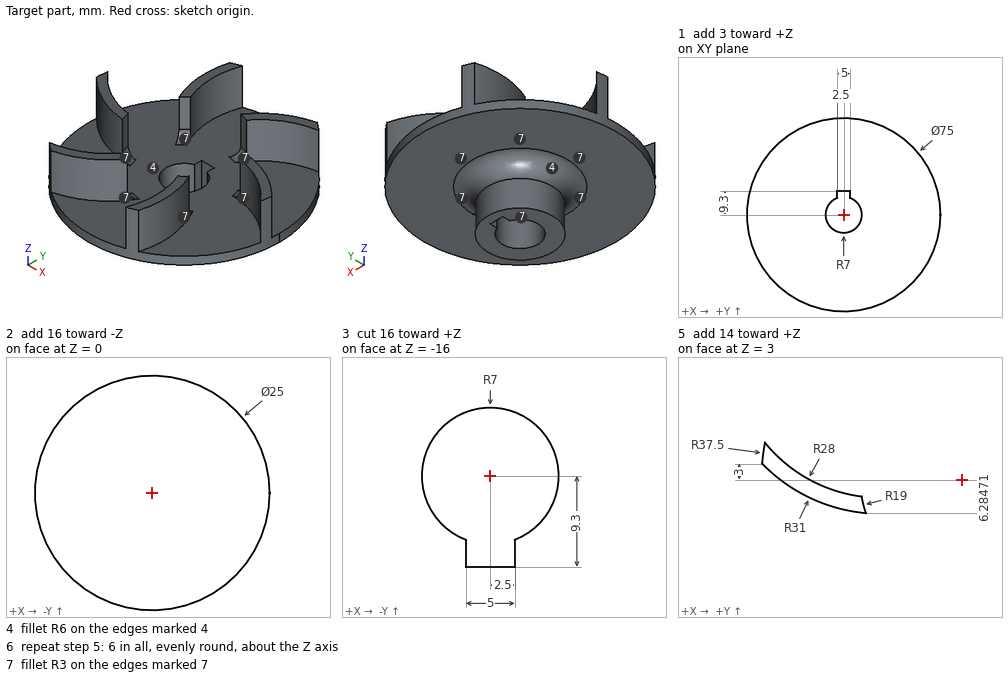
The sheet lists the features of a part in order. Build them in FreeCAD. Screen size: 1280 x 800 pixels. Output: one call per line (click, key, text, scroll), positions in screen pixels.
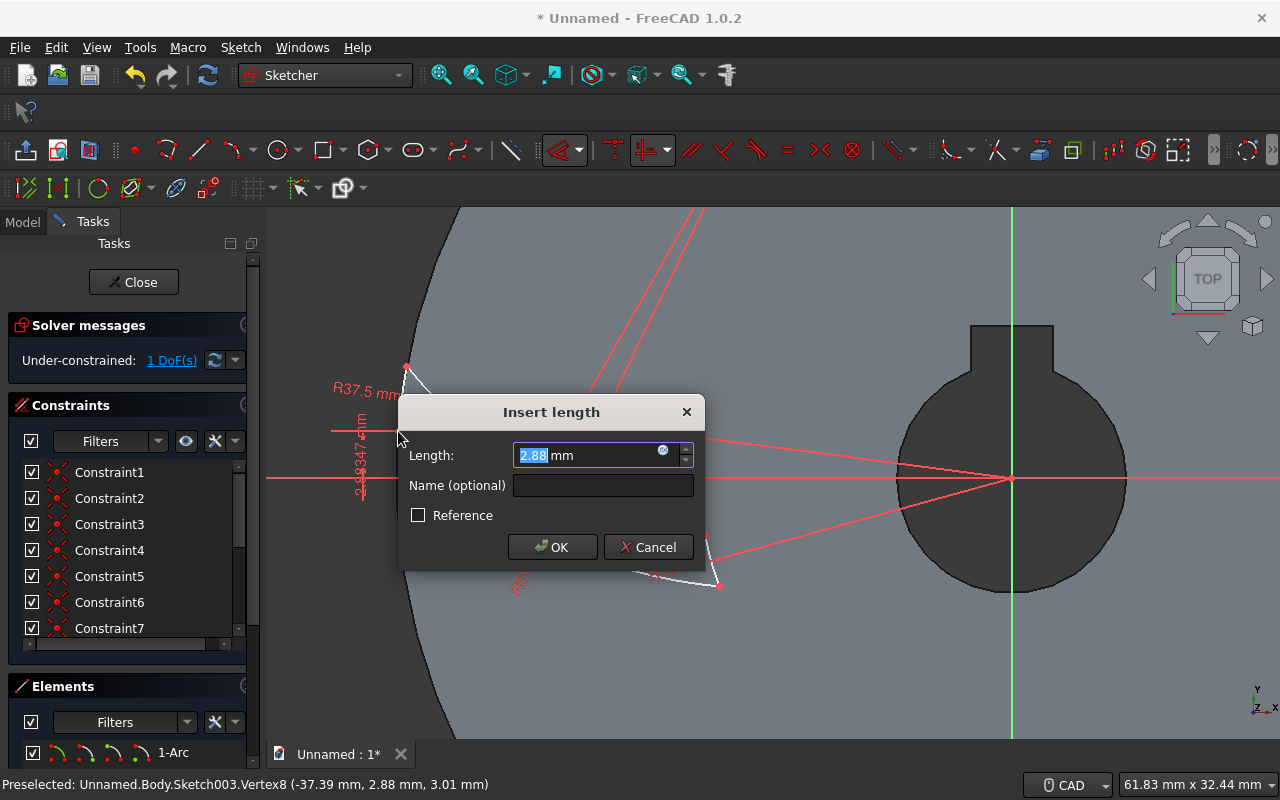
text(3)
key(Return)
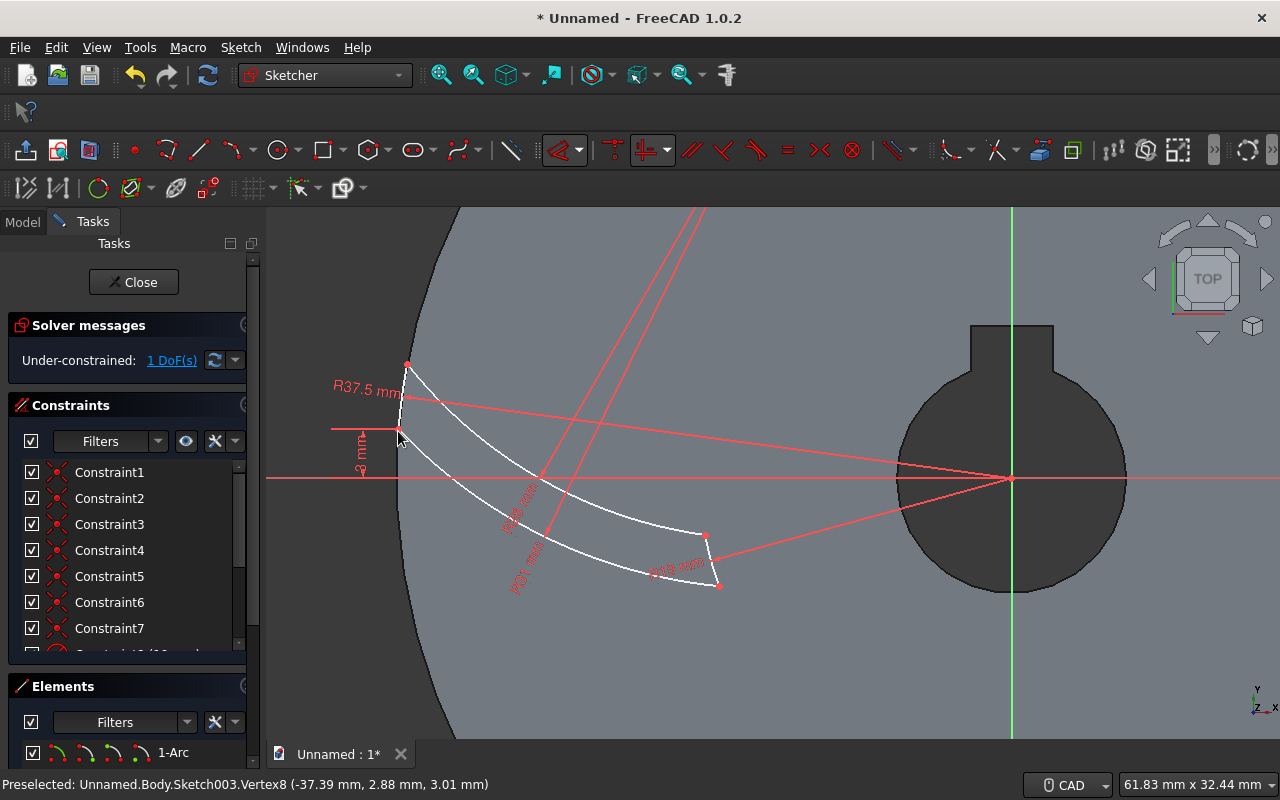
click(719, 586)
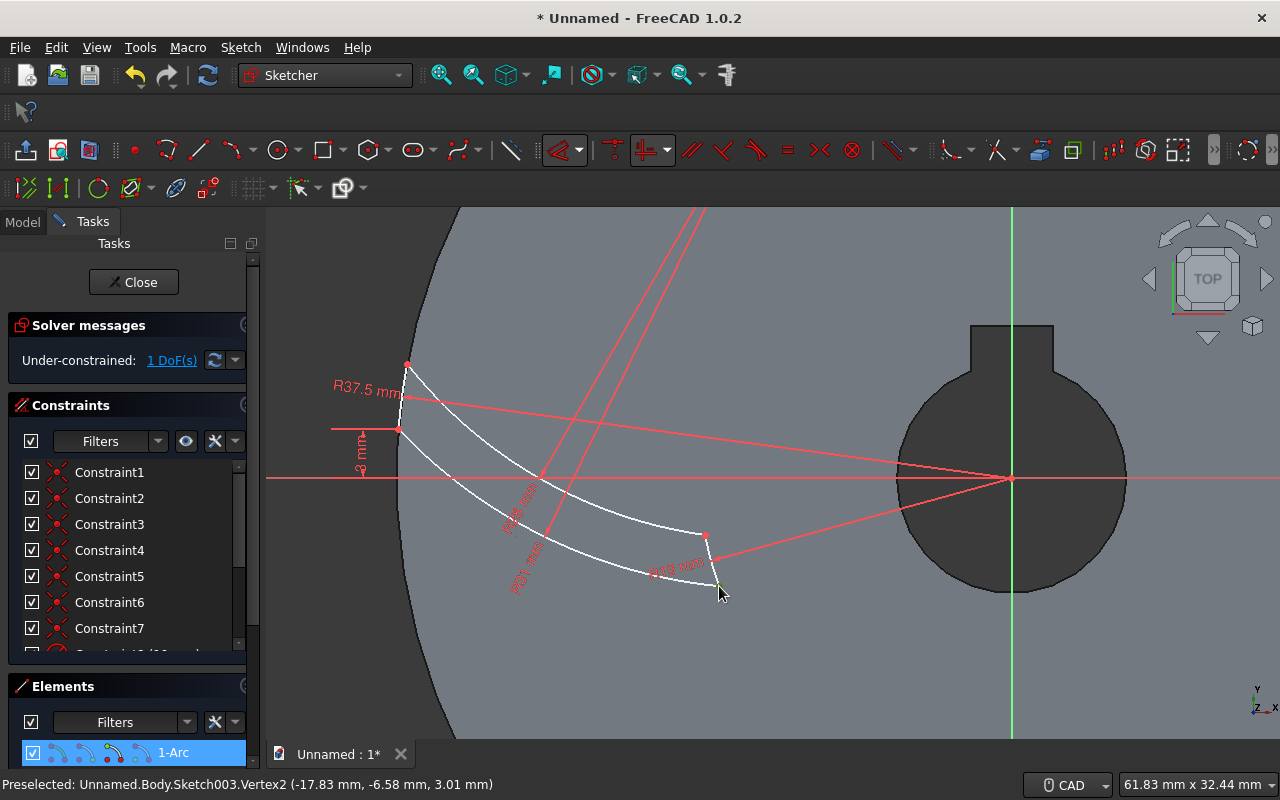
key(i)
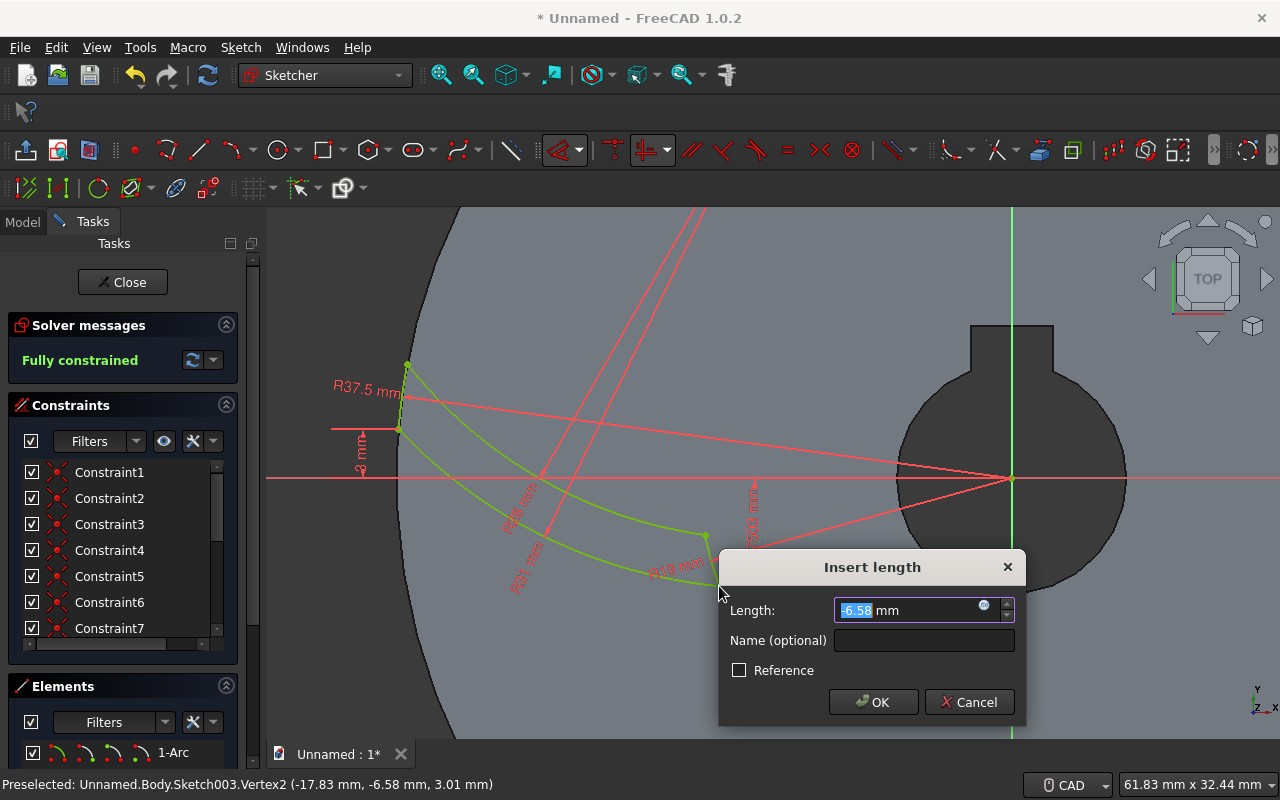
text(-6.28471)
key(Return)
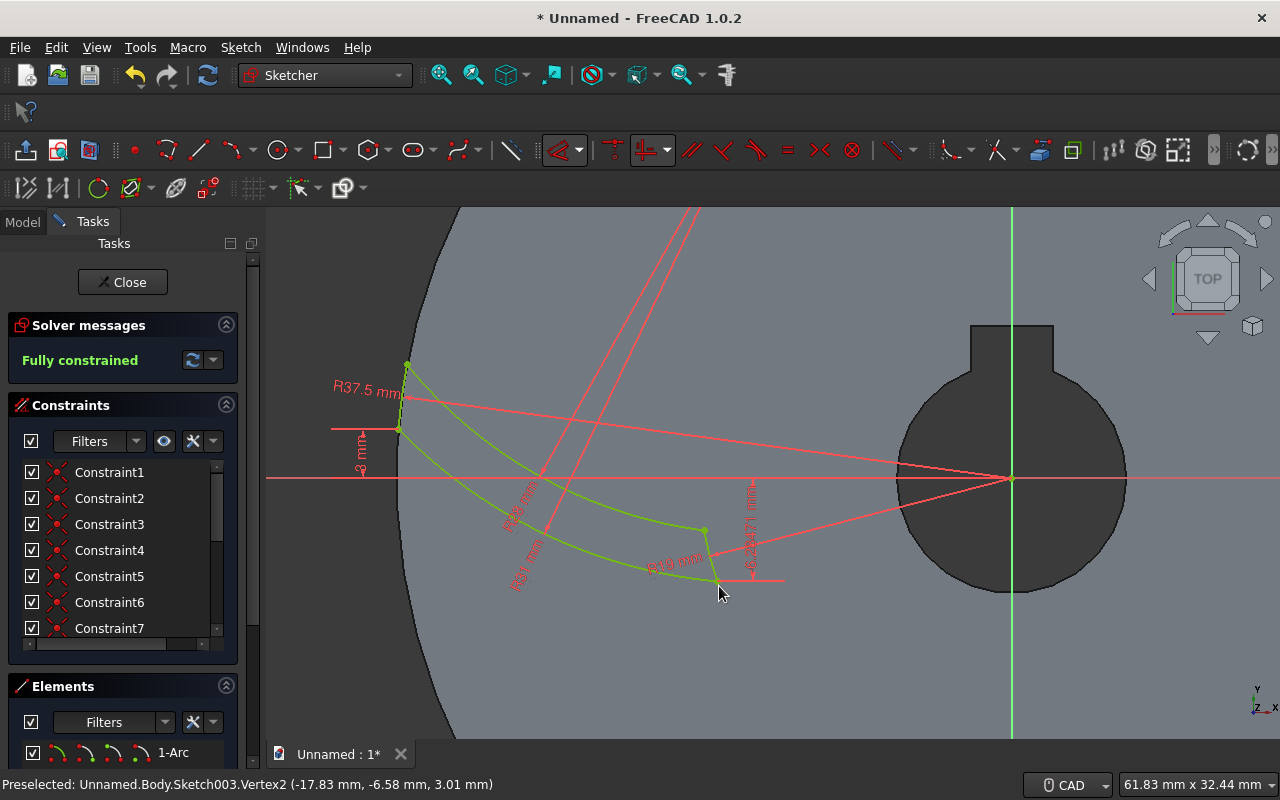
click(123, 282)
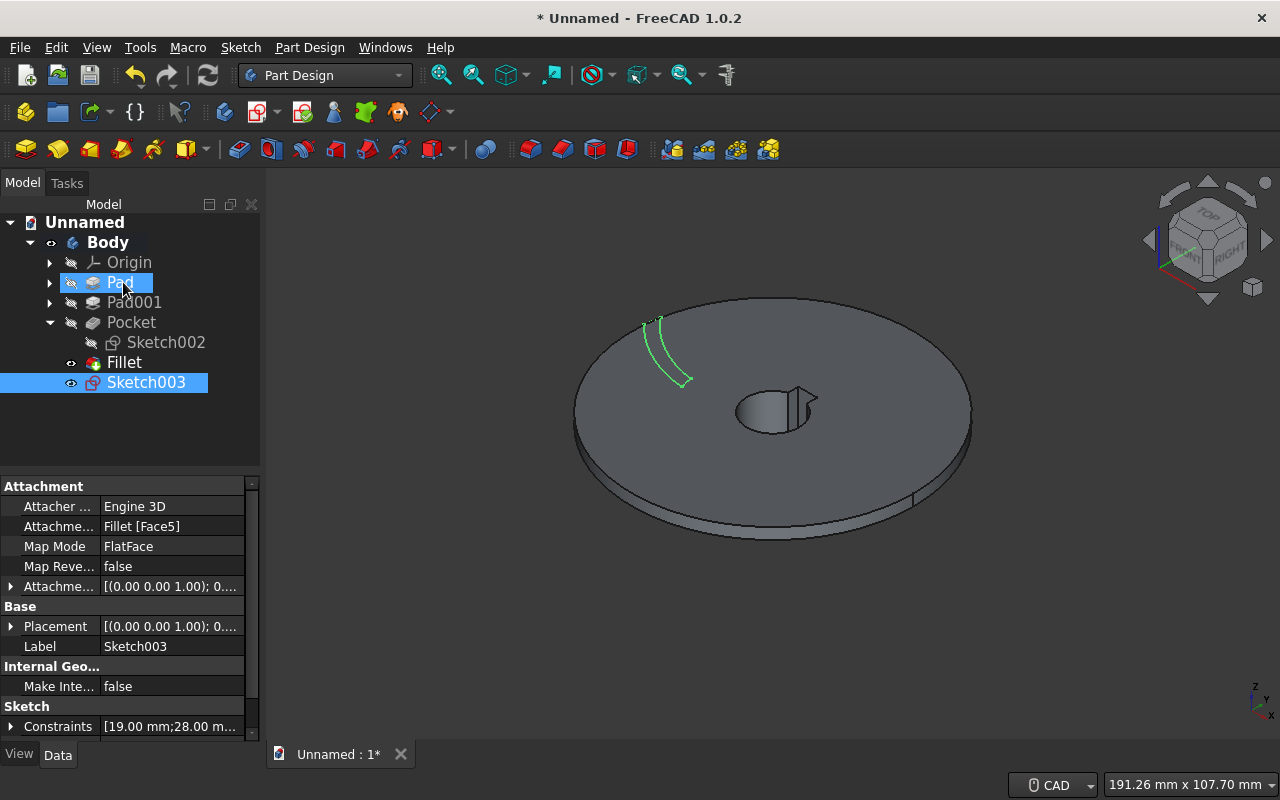
click(26, 150)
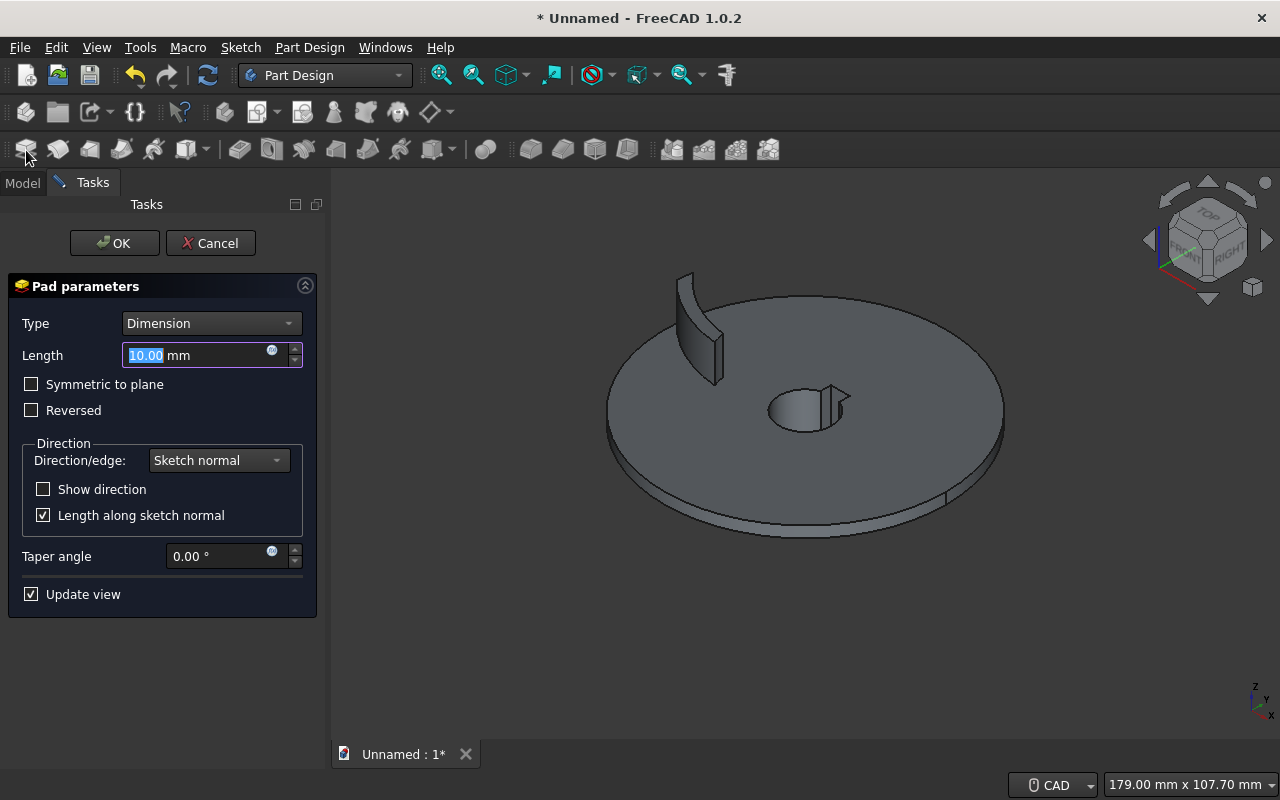
text(14)
key(Tab)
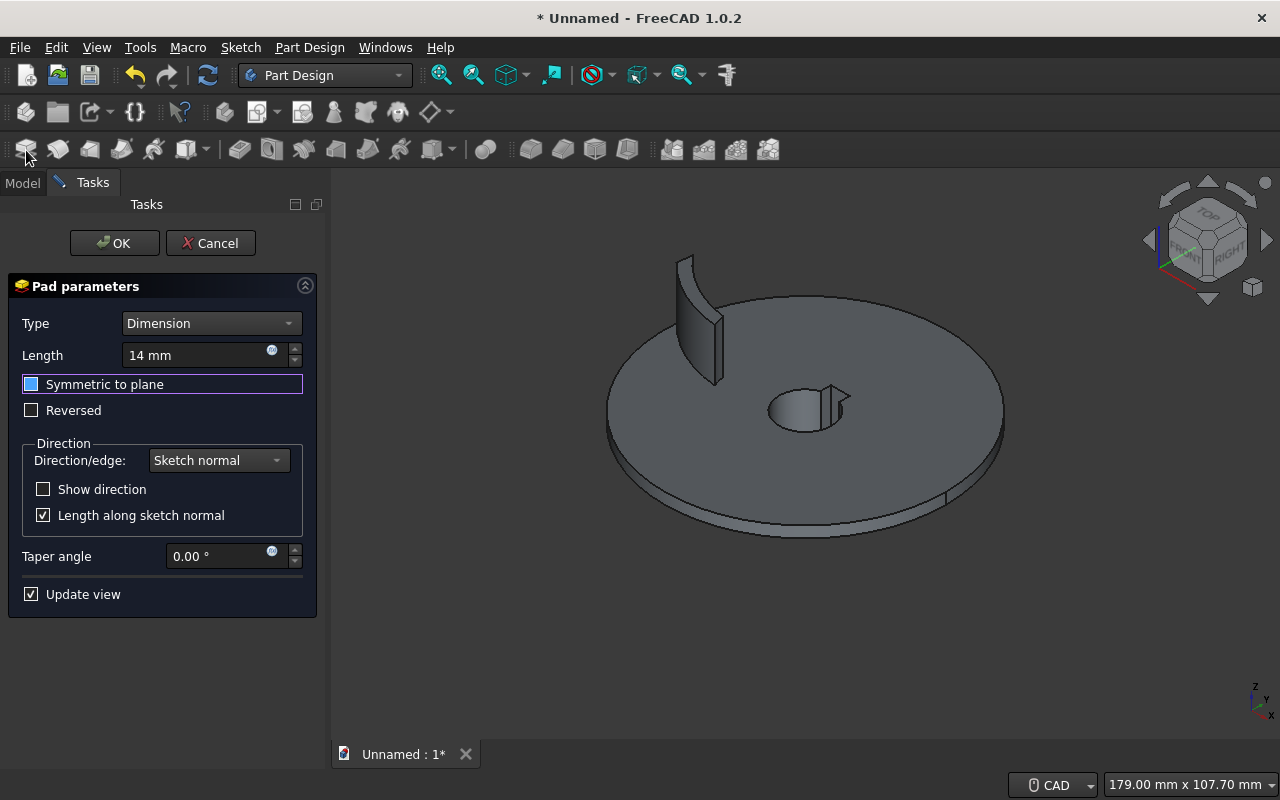
click(115, 243)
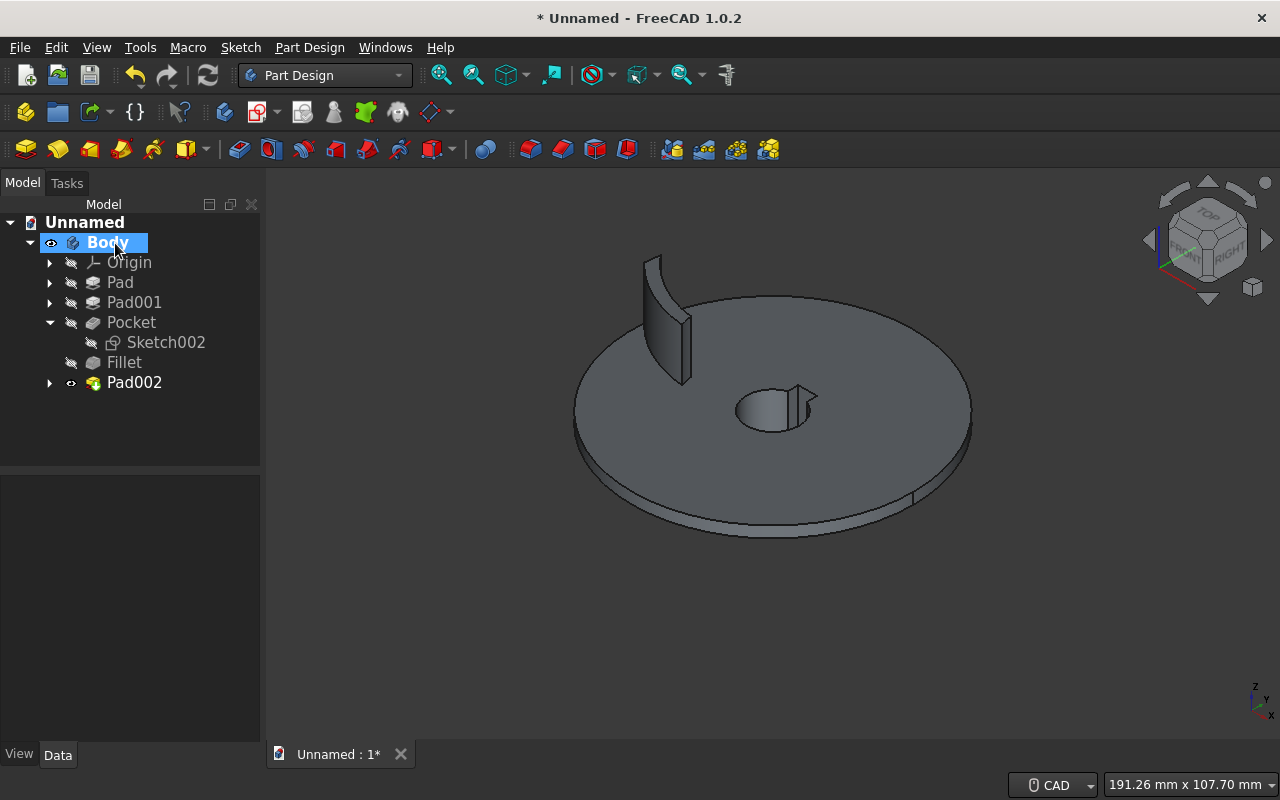
click(116, 383)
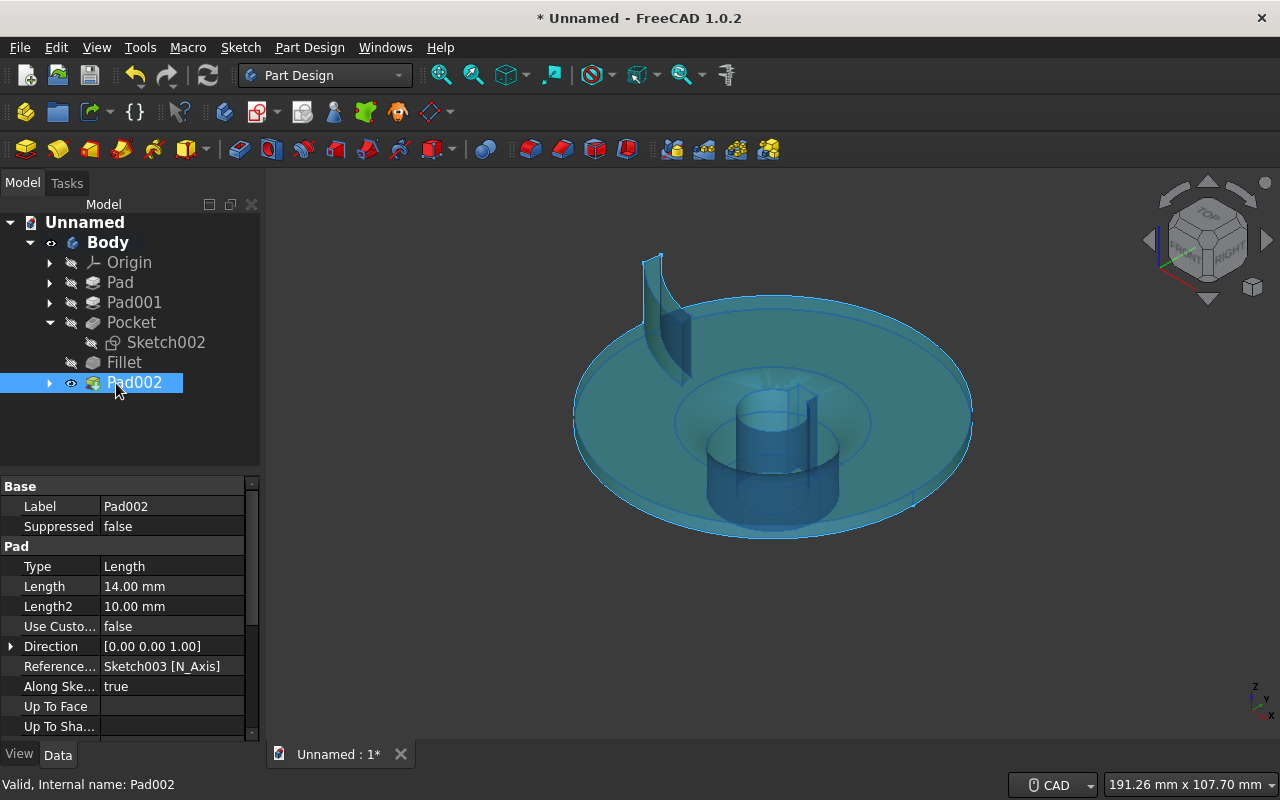
click(736, 150)